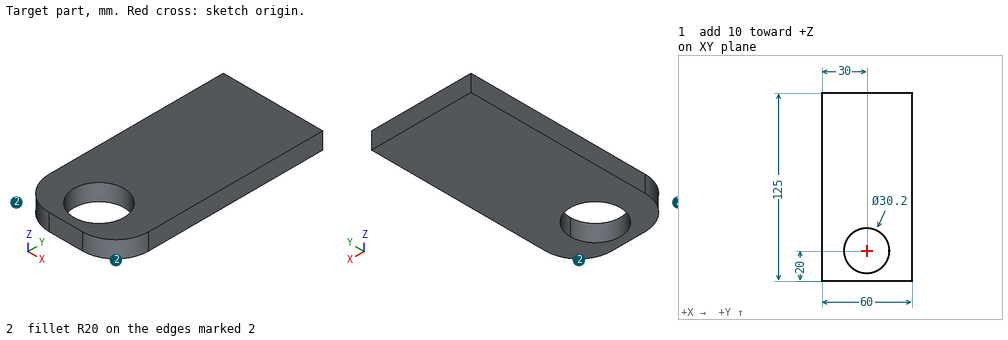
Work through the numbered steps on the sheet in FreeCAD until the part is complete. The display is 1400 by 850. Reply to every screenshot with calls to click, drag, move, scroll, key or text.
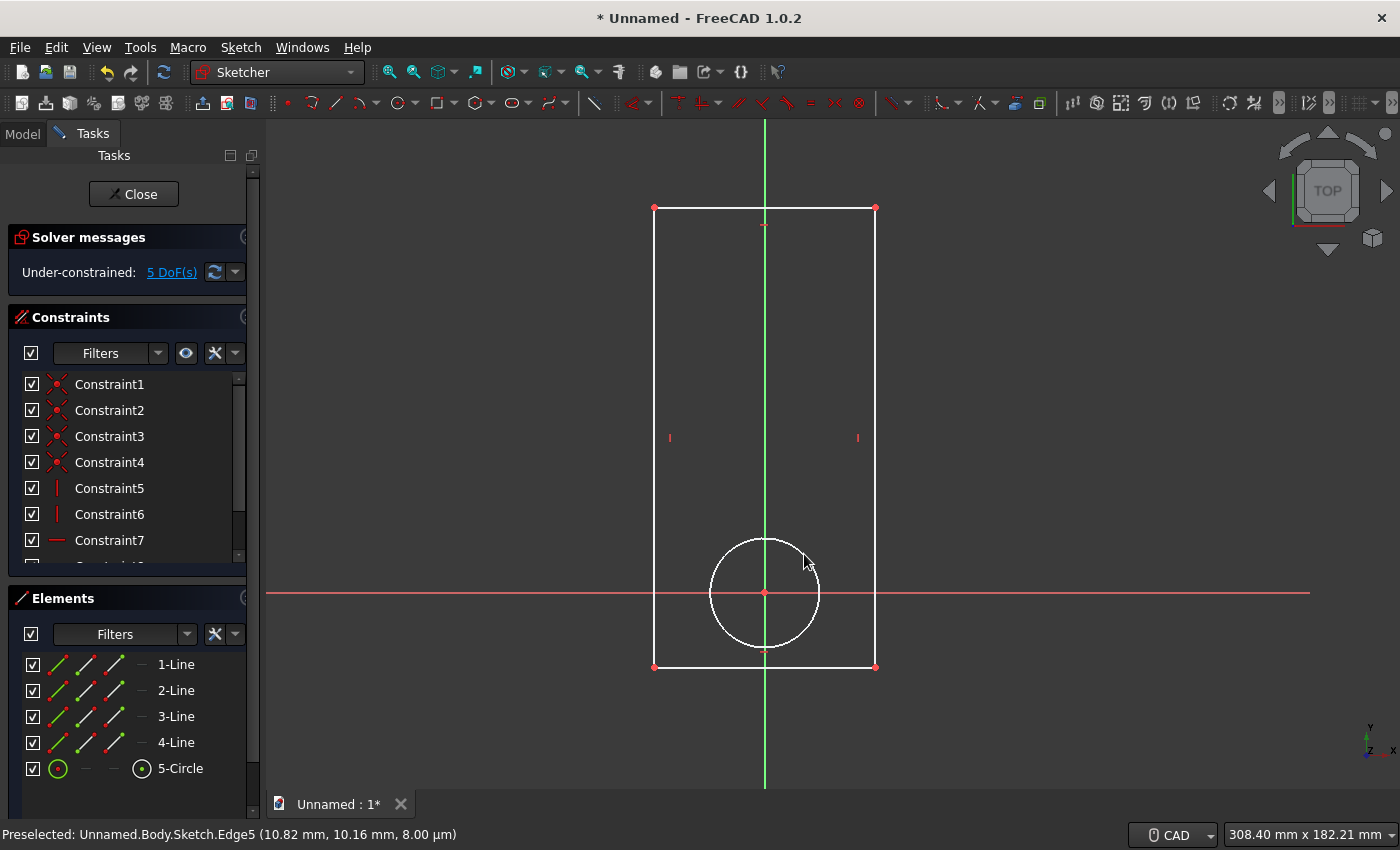
click(632, 104)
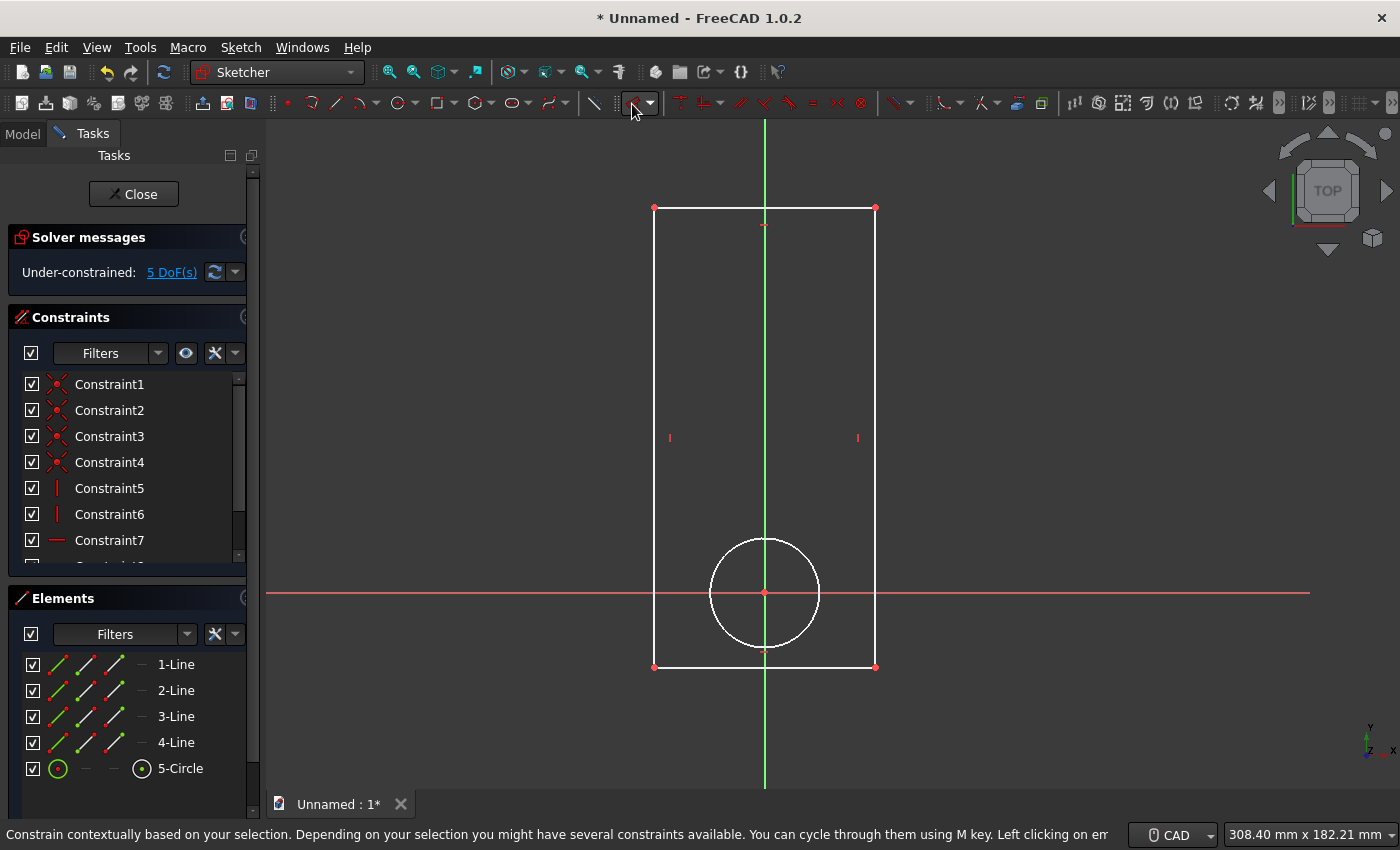
click(803, 554)
click(825, 531)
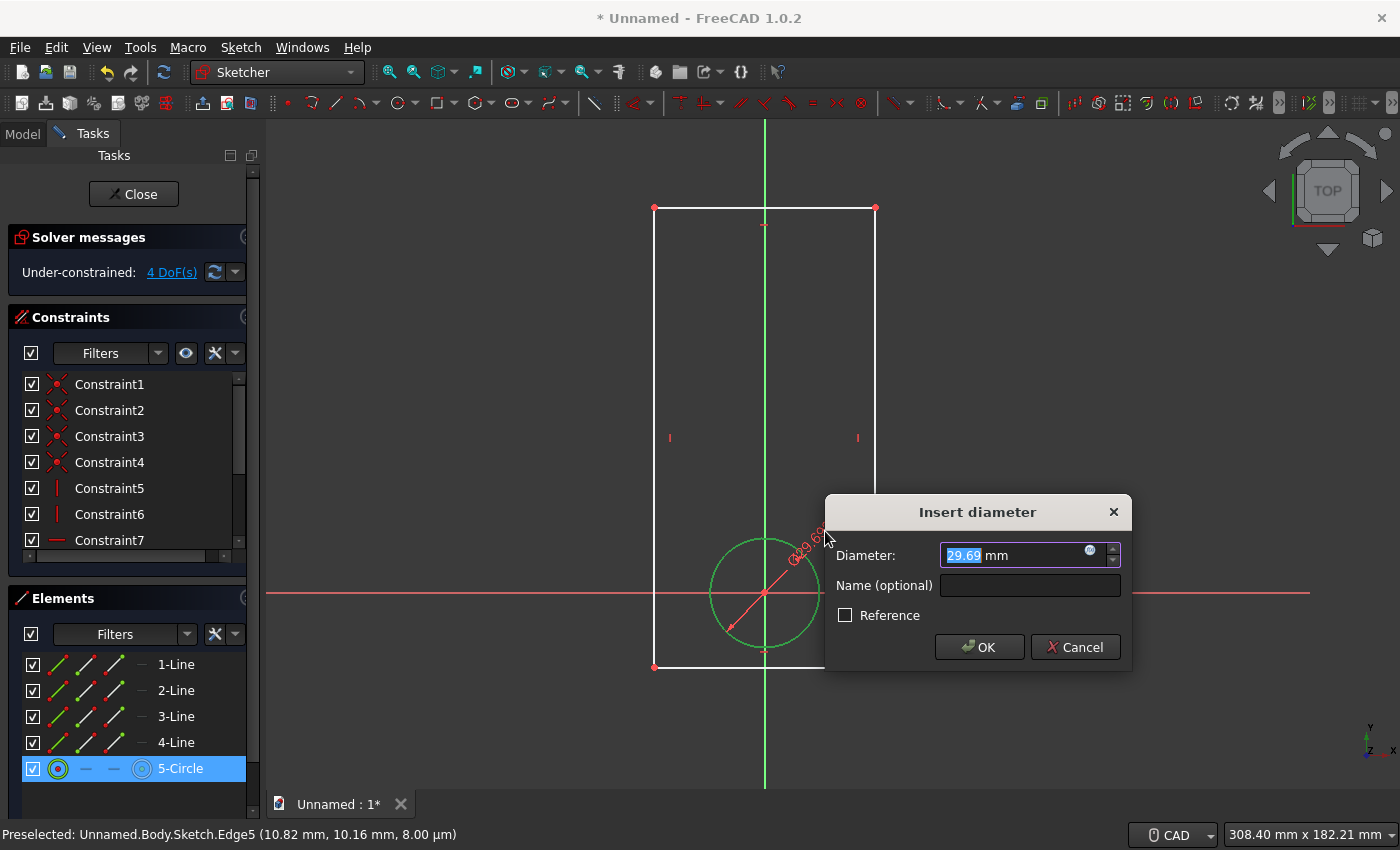
text(30.2)
key(Return)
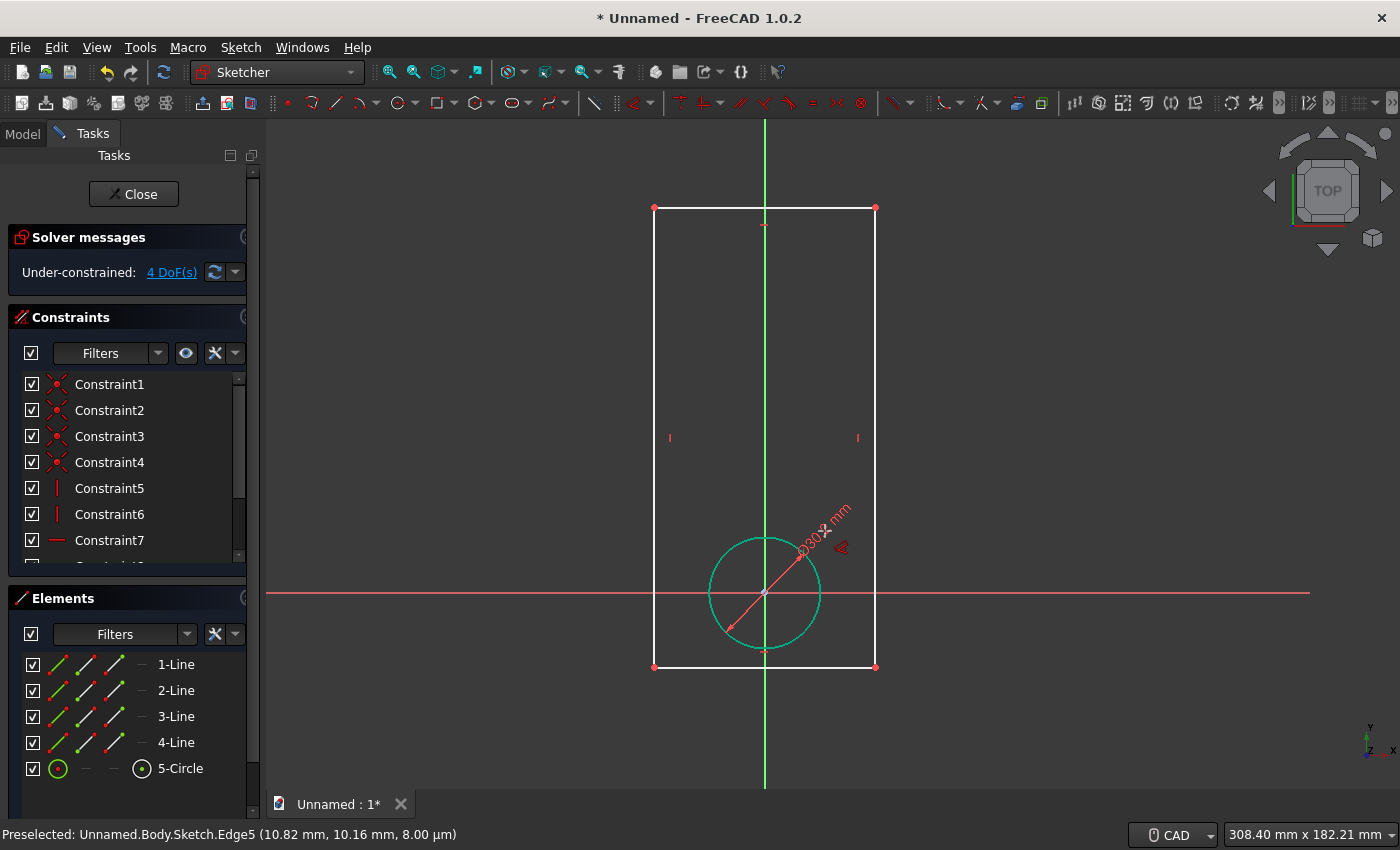
click(720, 668)
click(714, 702)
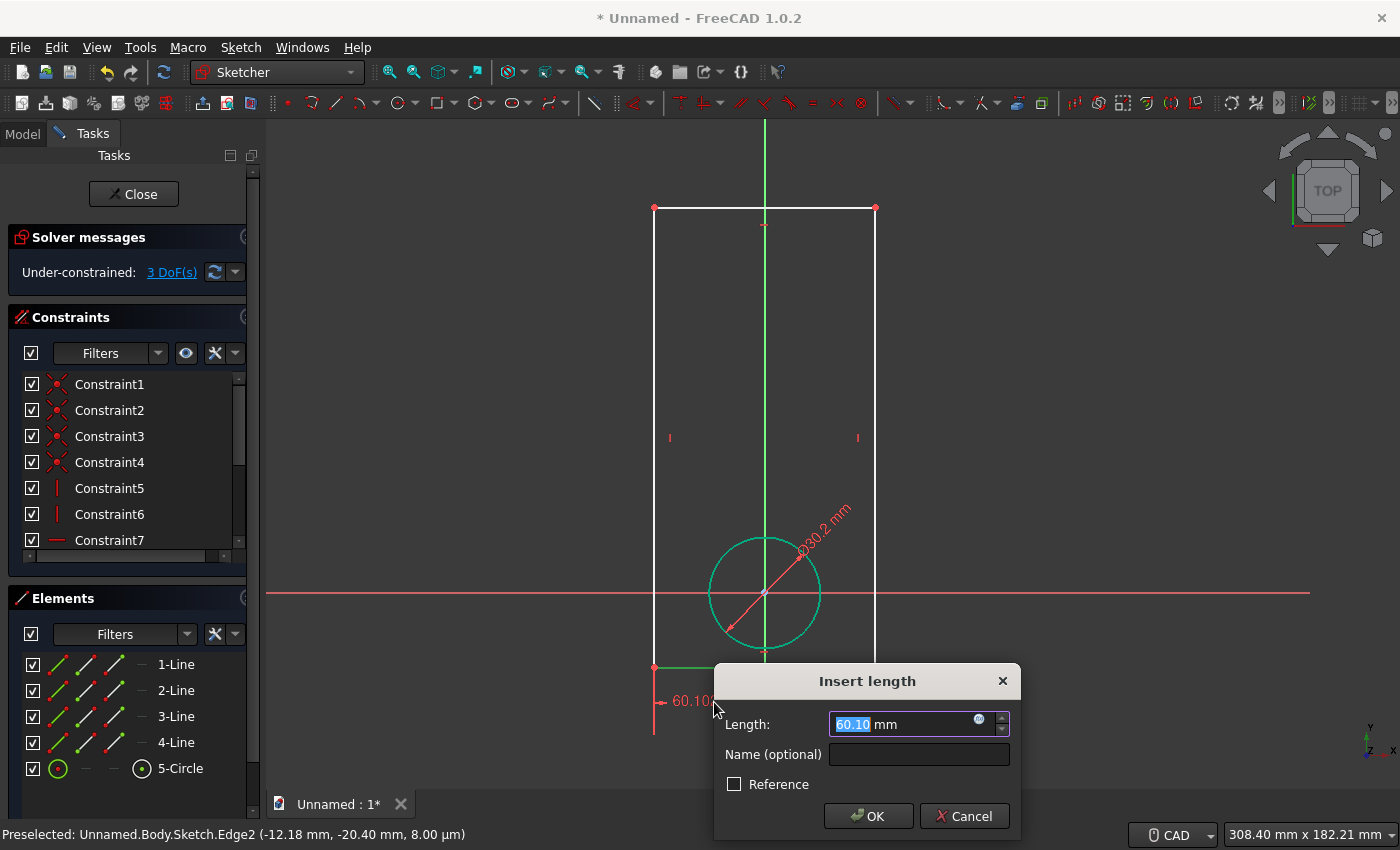
text(60)
key(Return)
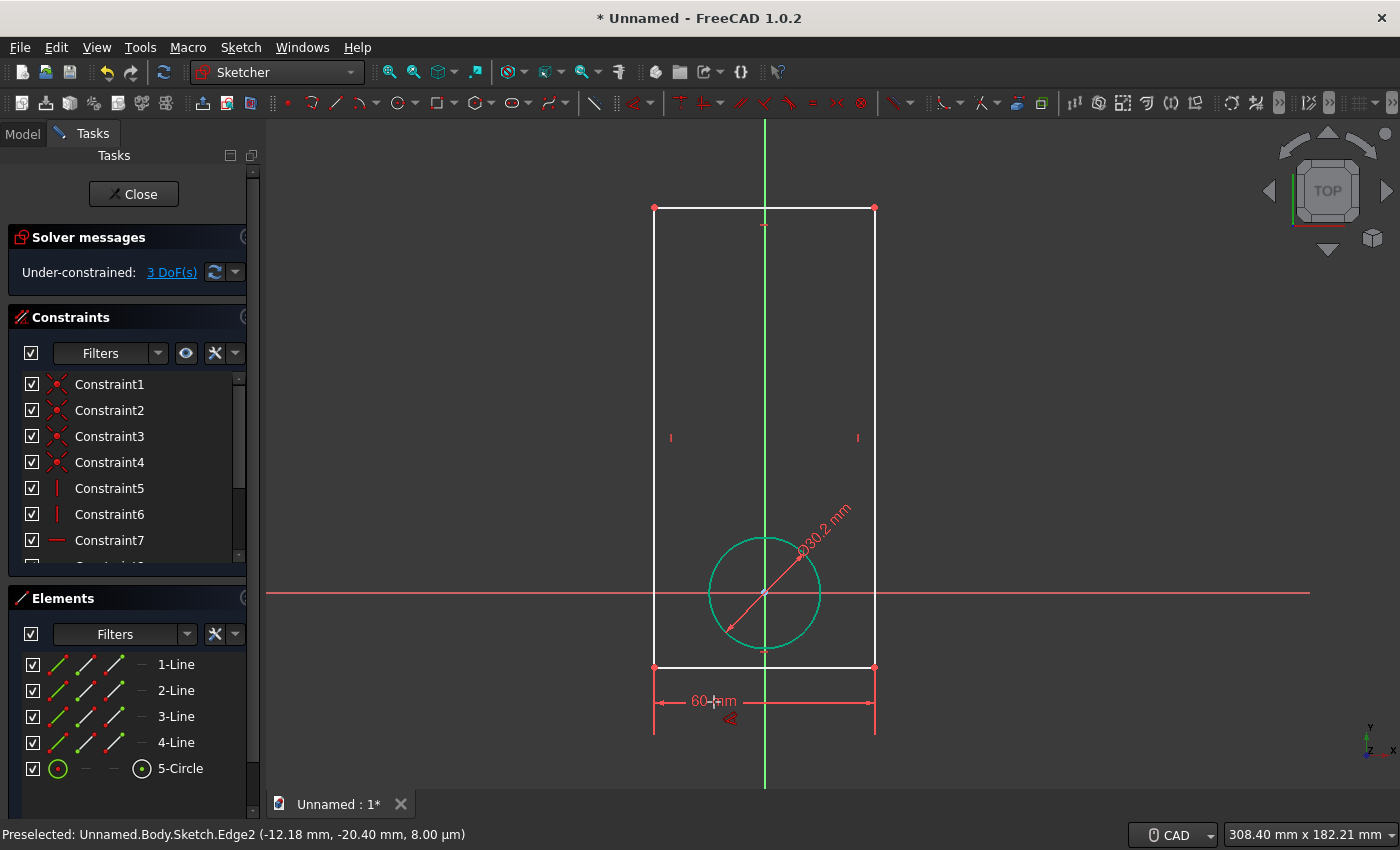
click(654, 346)
click(620, 438)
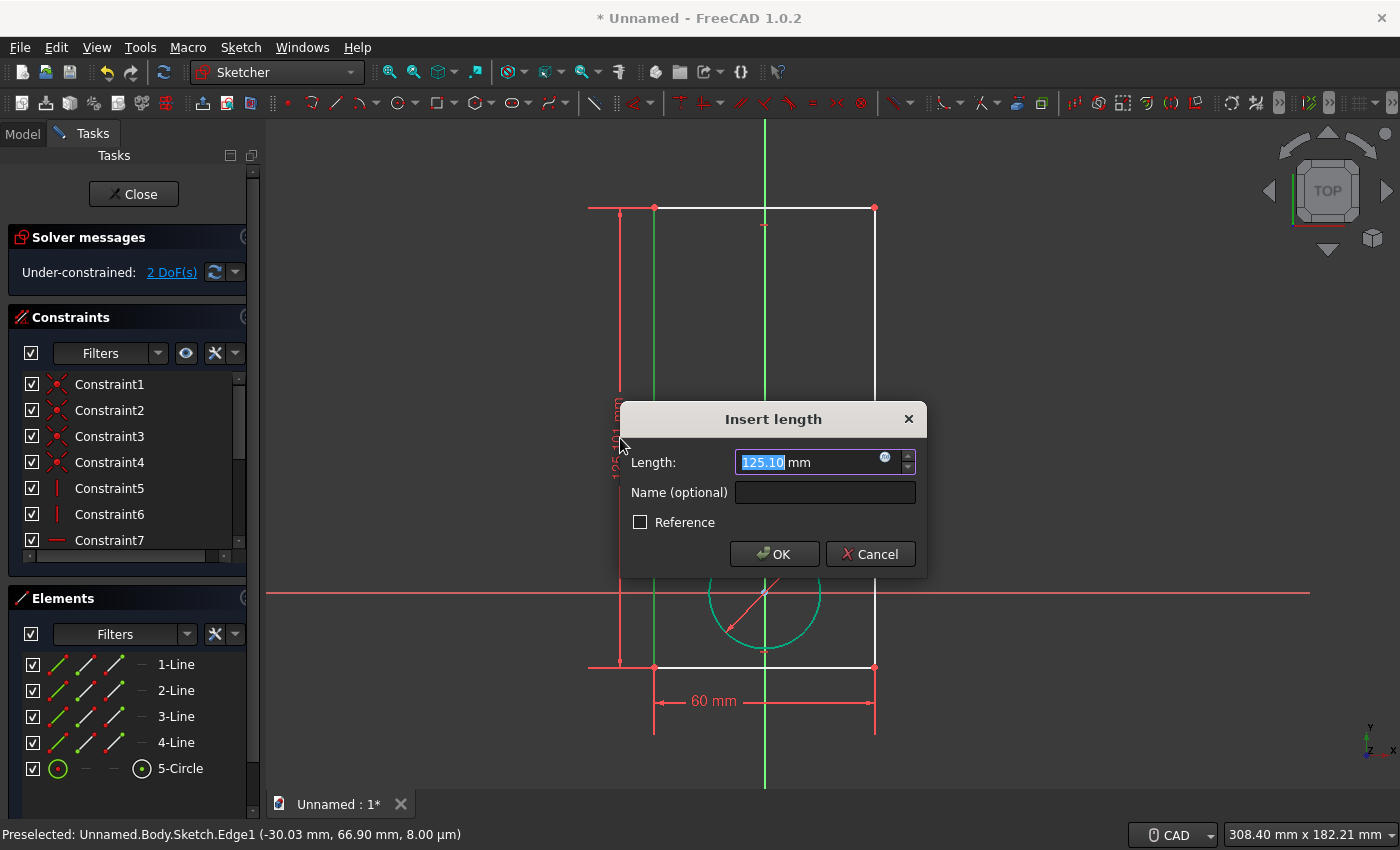
text(125)
key(Return)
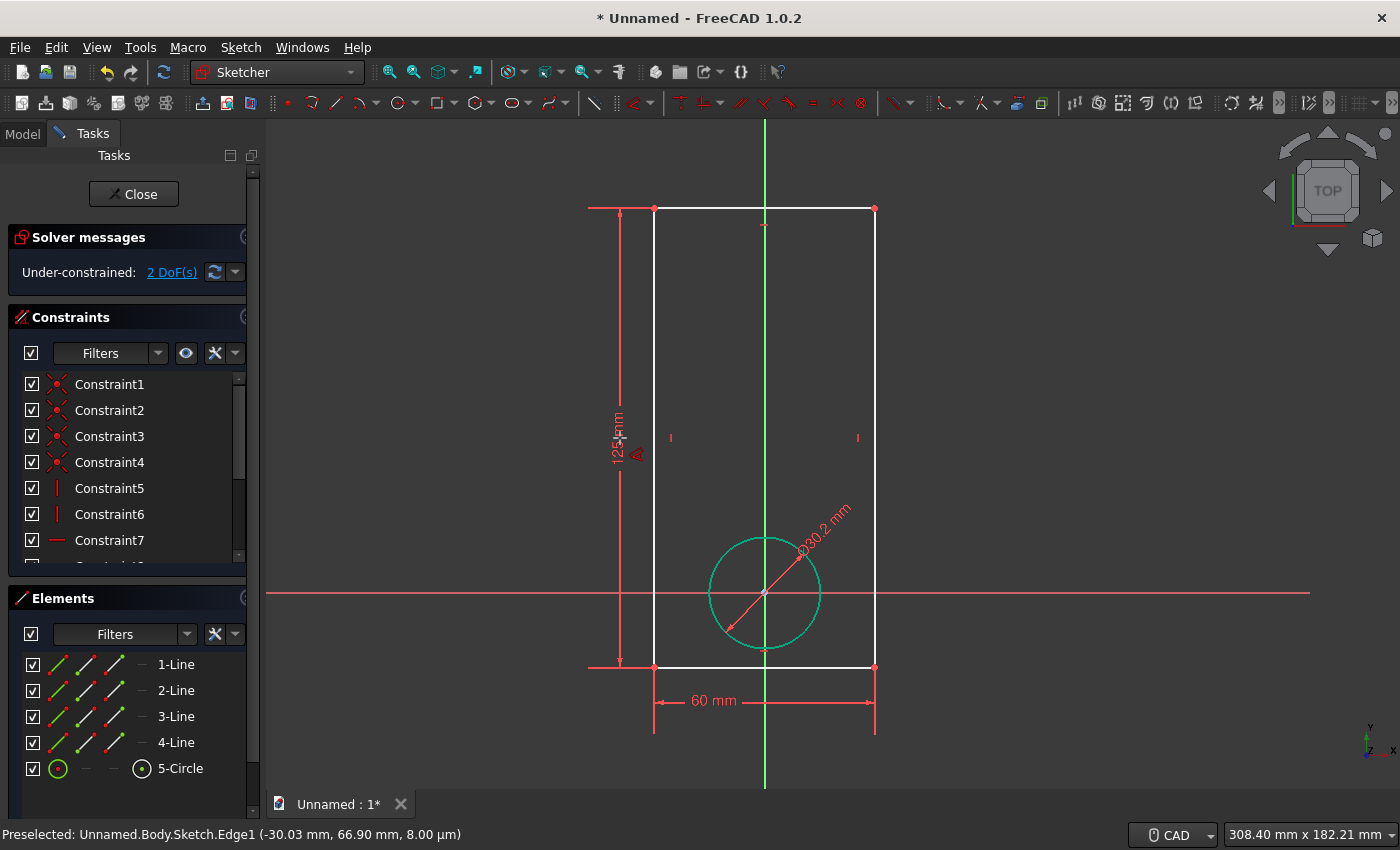
click(654, 208)
click(710, 174)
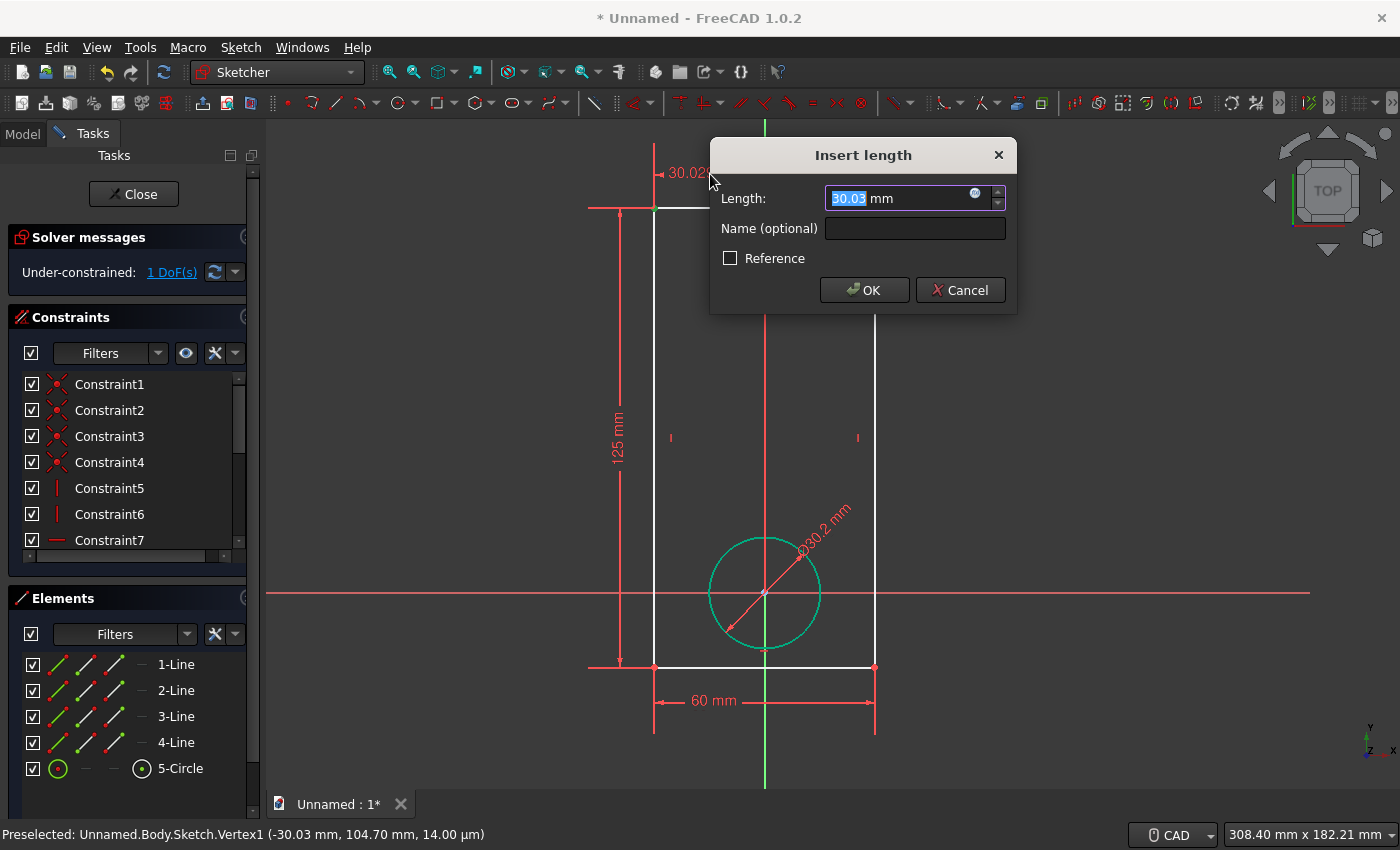
text(30)
key(Return)